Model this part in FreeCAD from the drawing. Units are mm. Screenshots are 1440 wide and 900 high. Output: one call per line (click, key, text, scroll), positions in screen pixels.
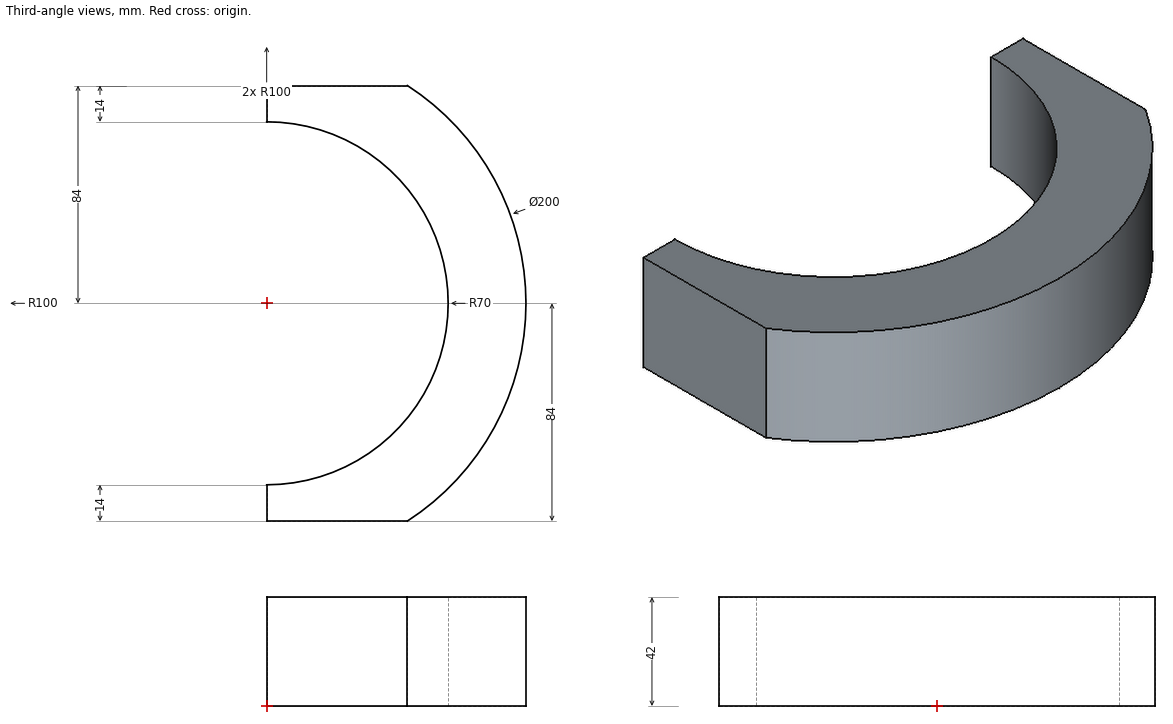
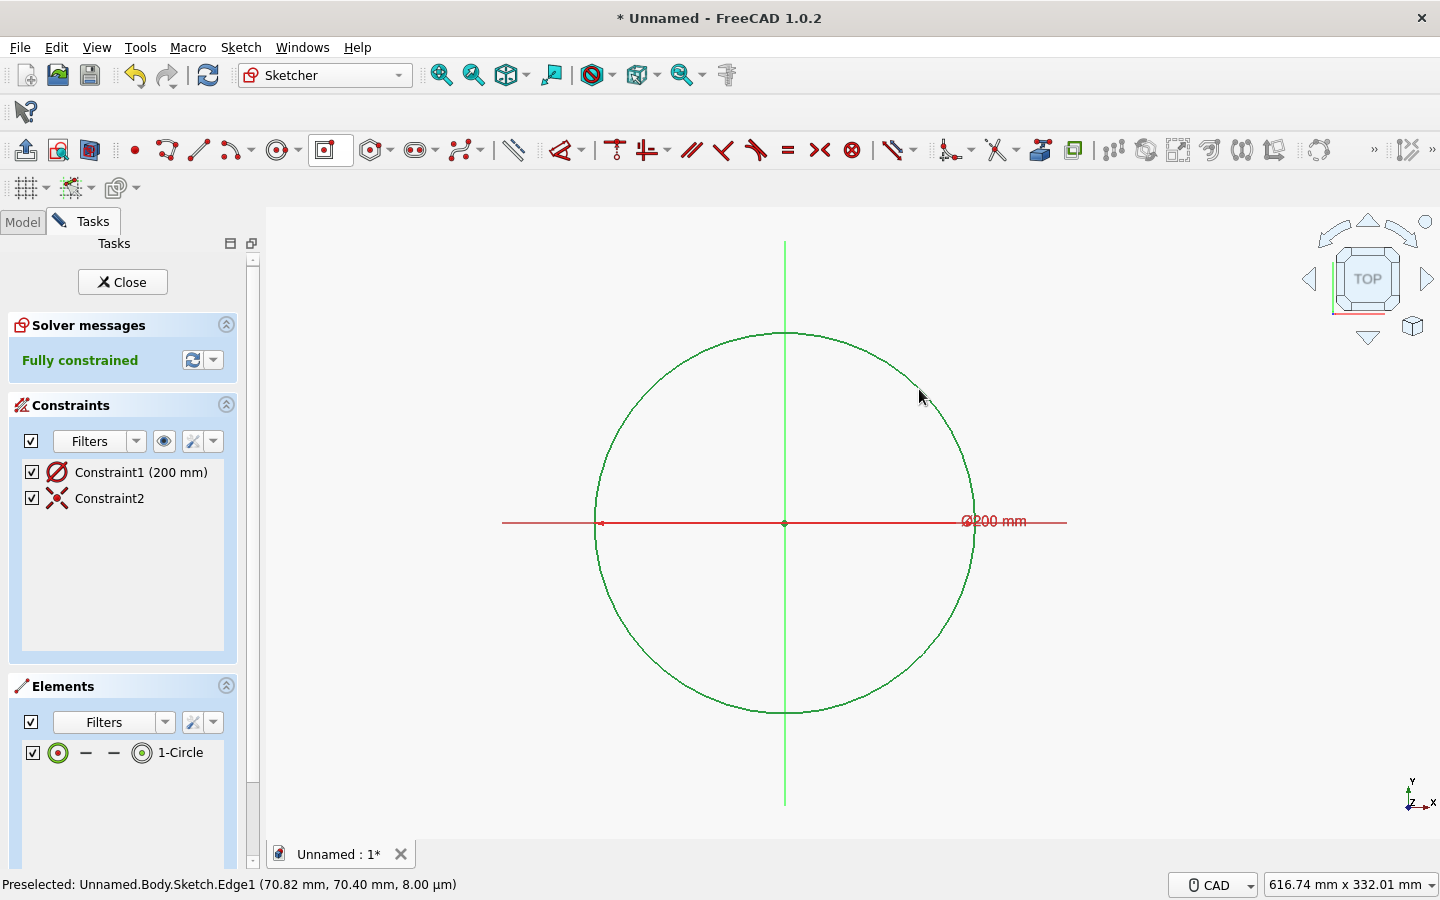
click(123, 282)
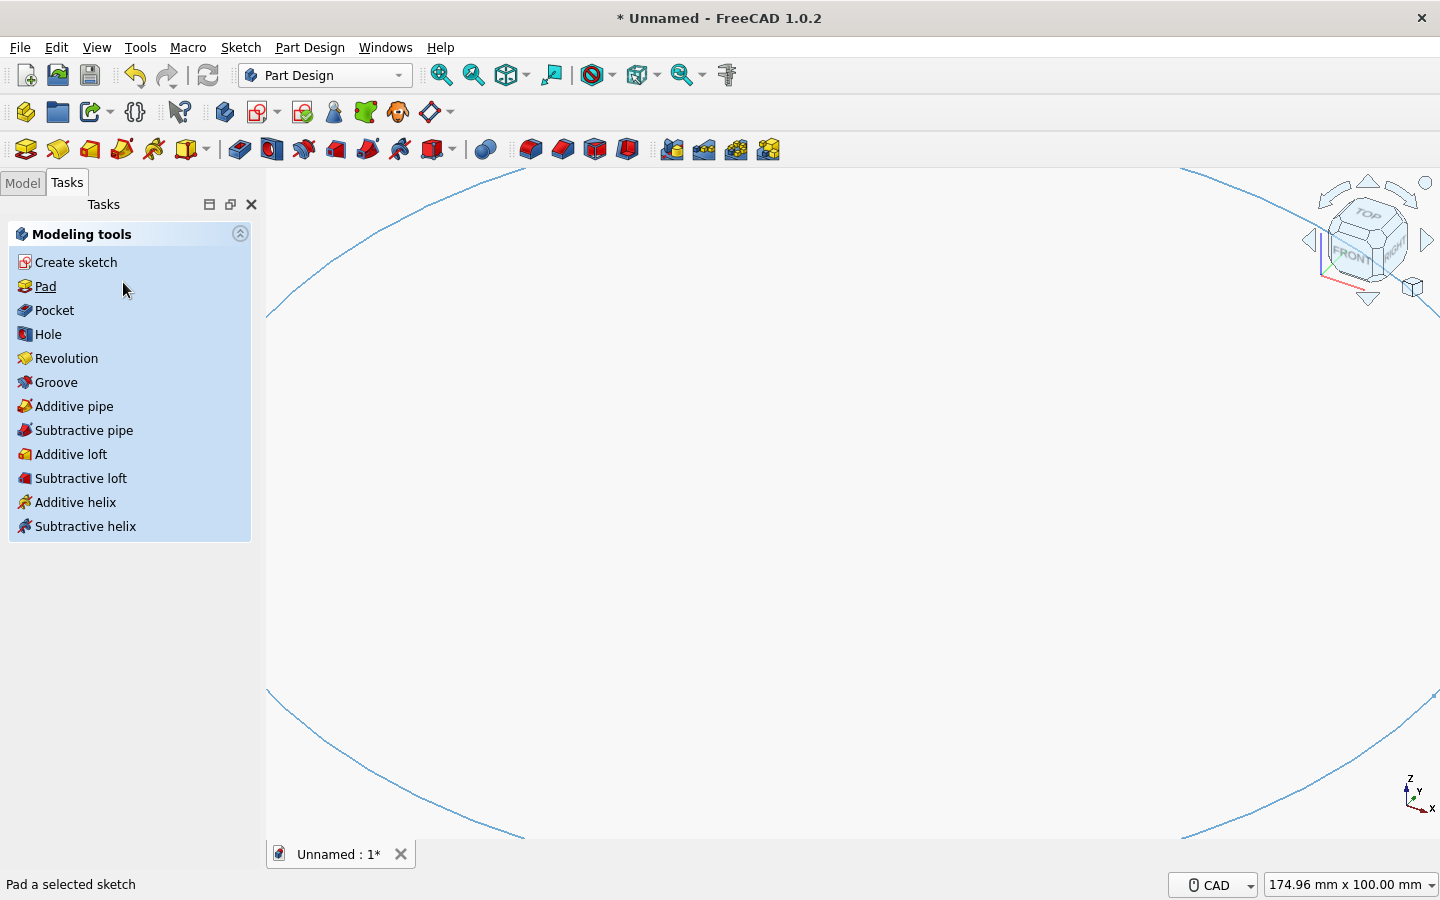
click(26, 150)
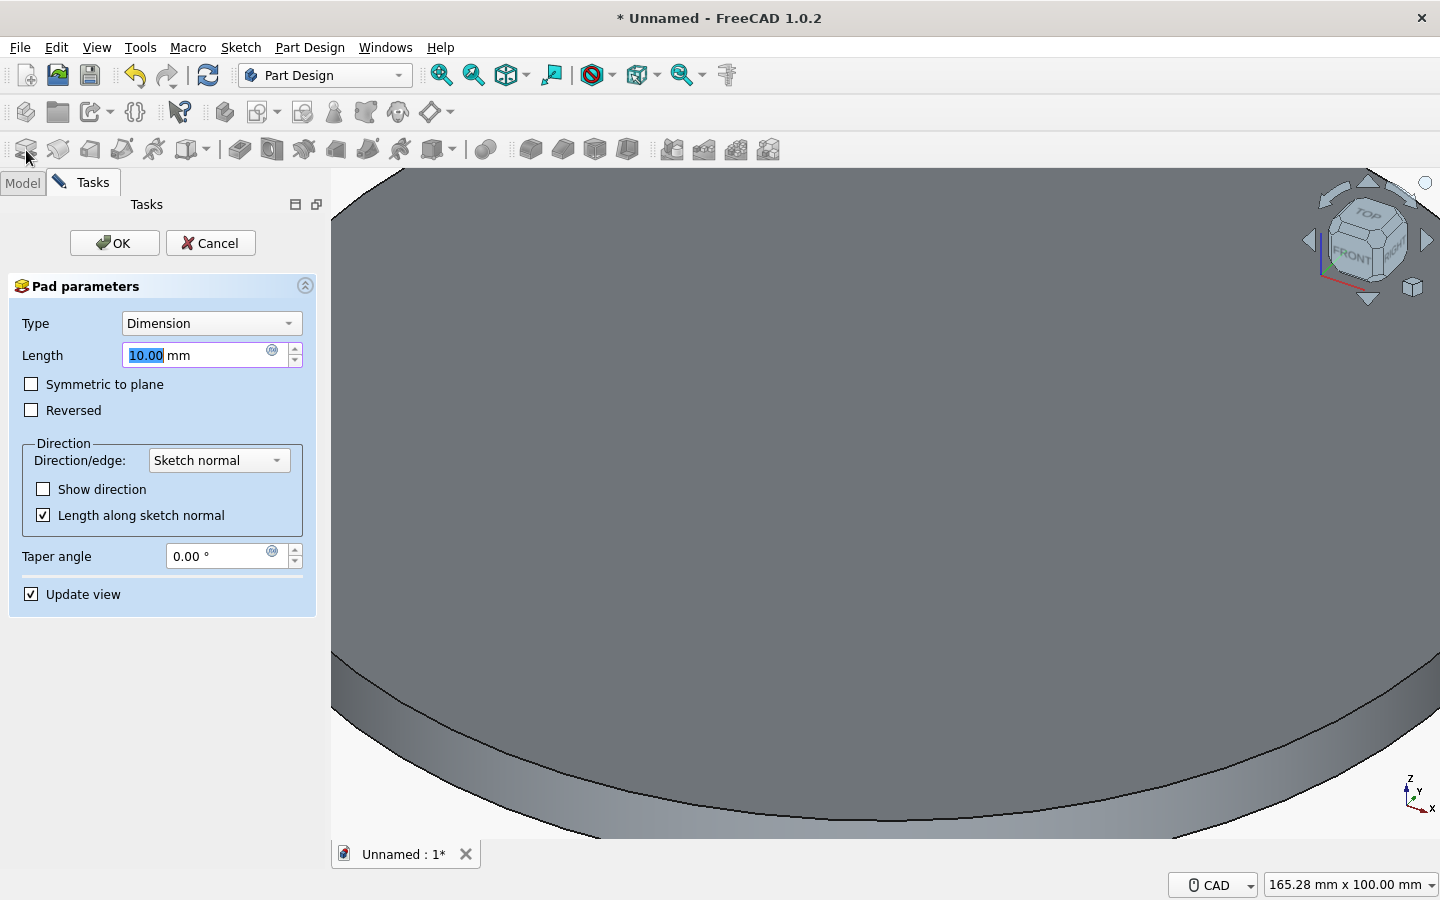
text(42)
key(Tab)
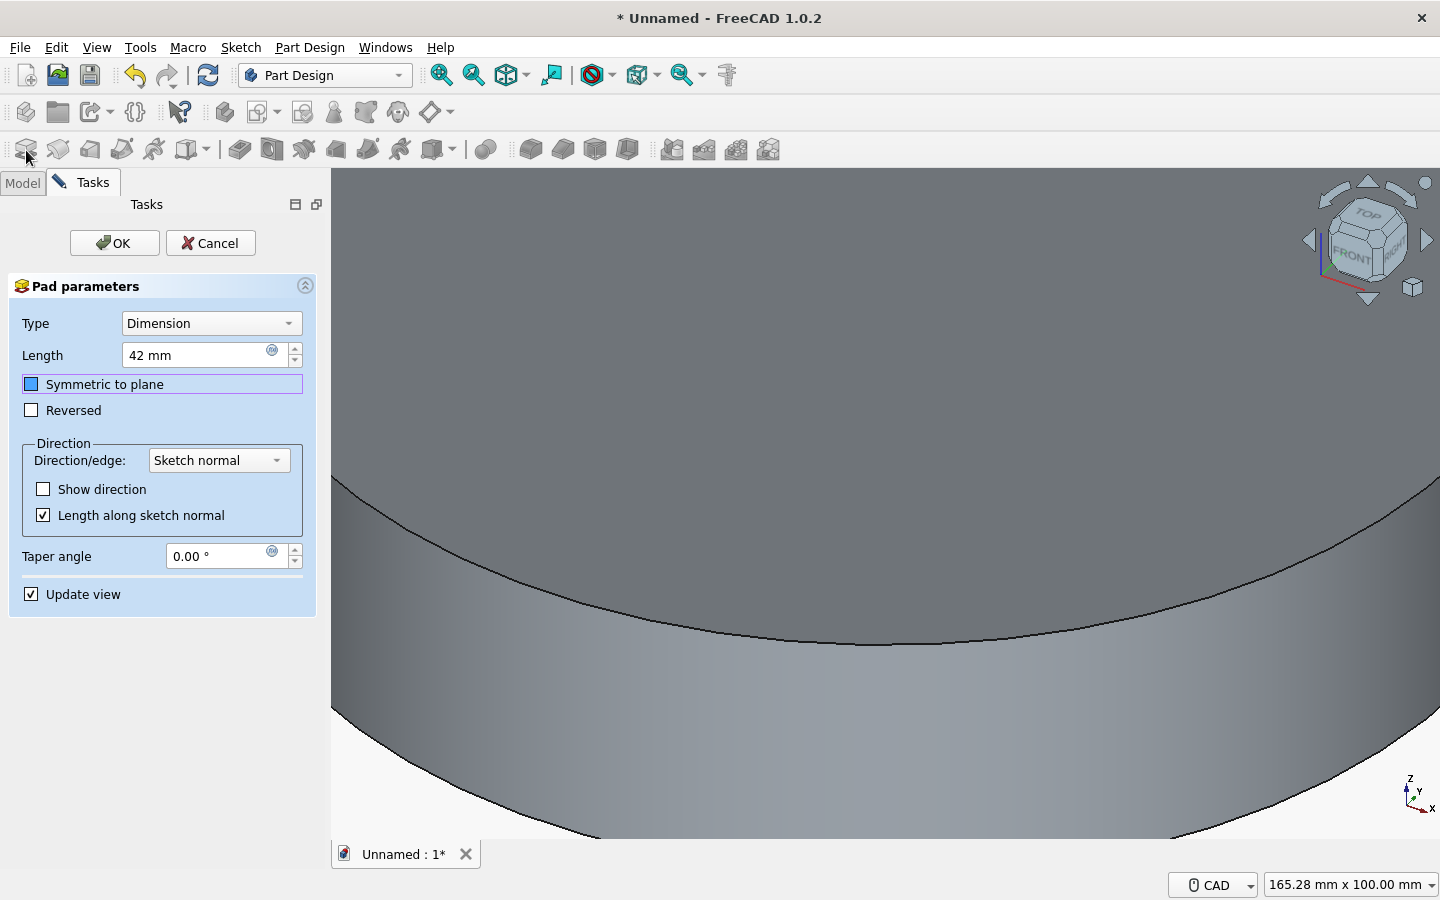
click(115, 243)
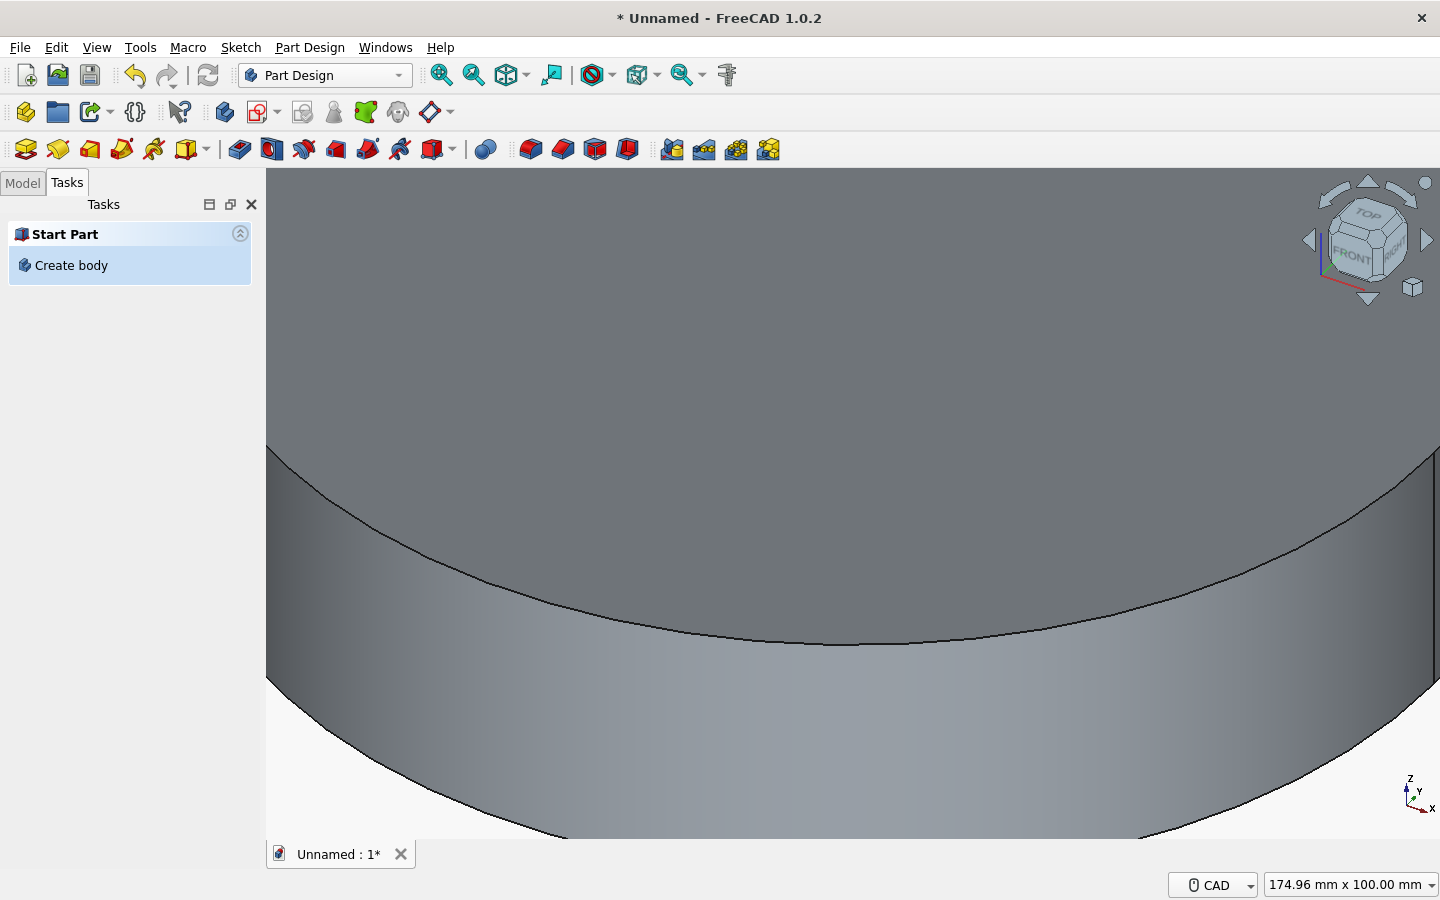
click(442, 76)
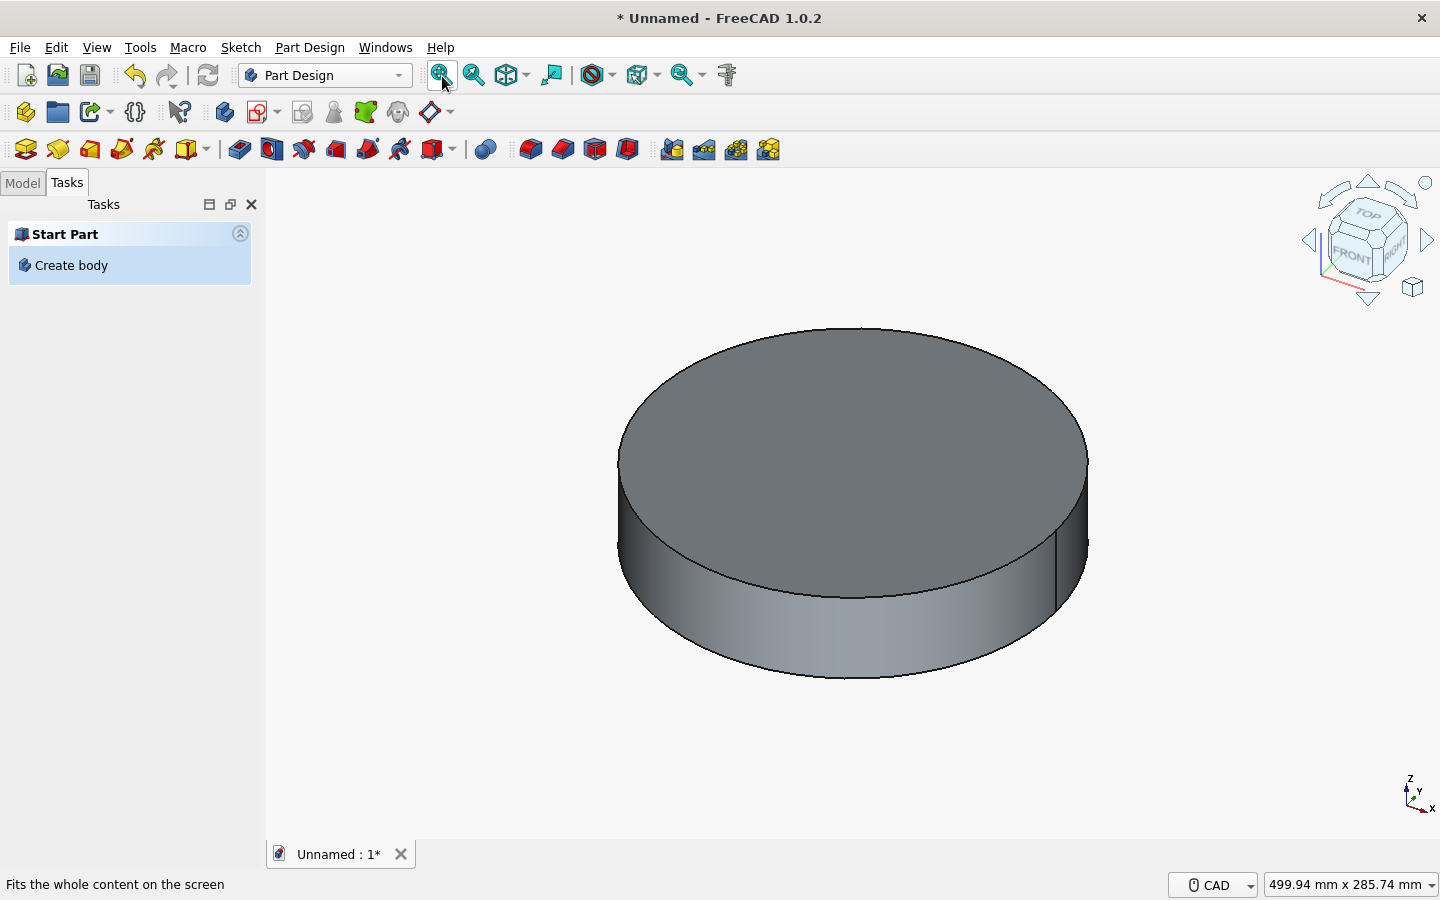
click(853, 462)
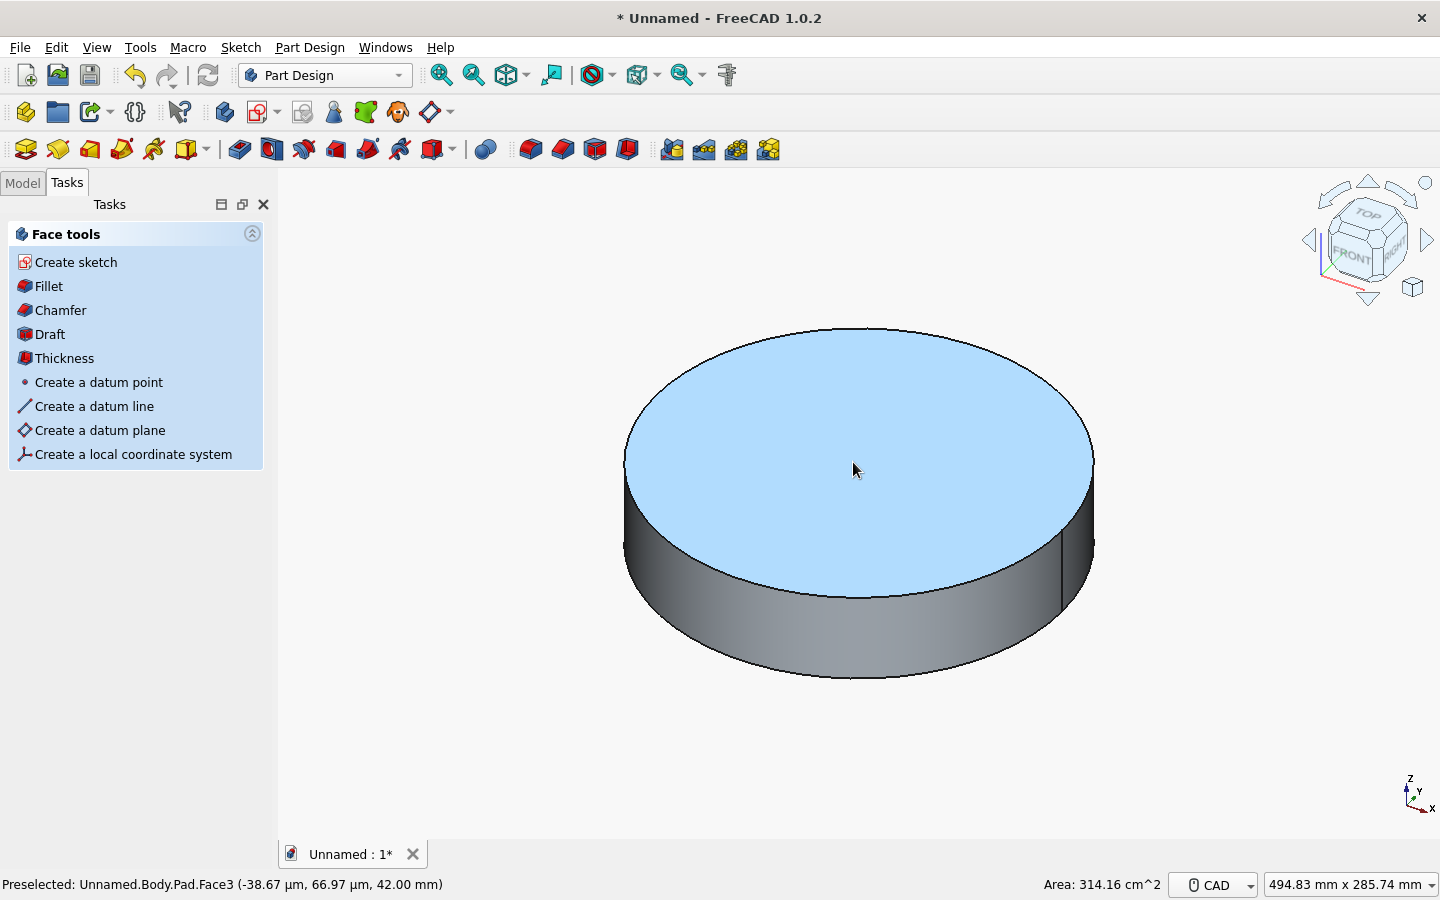
click(258, 112)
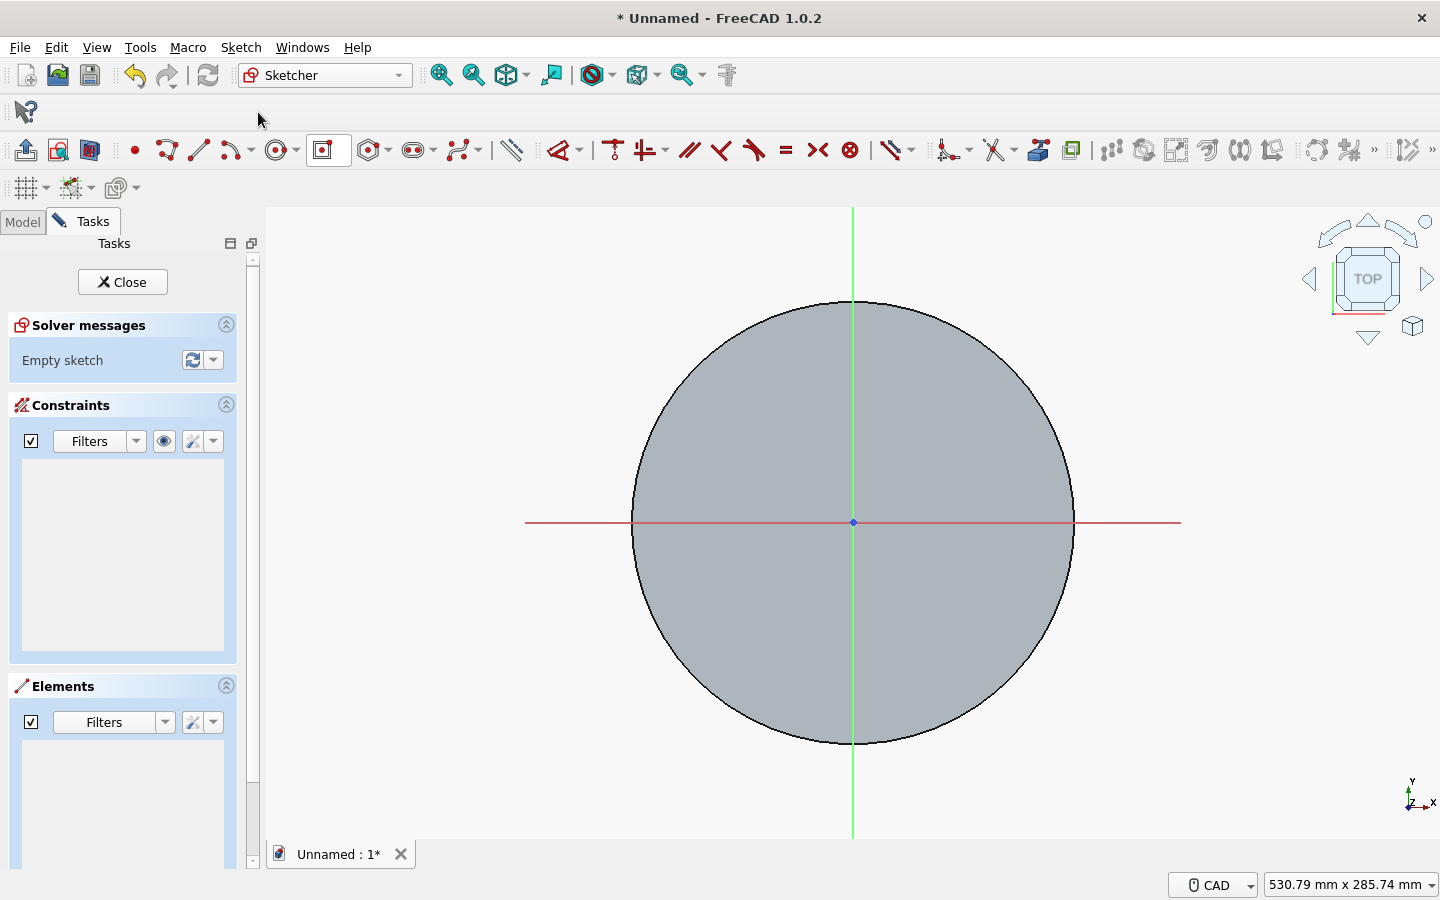
key(g)
key(l)